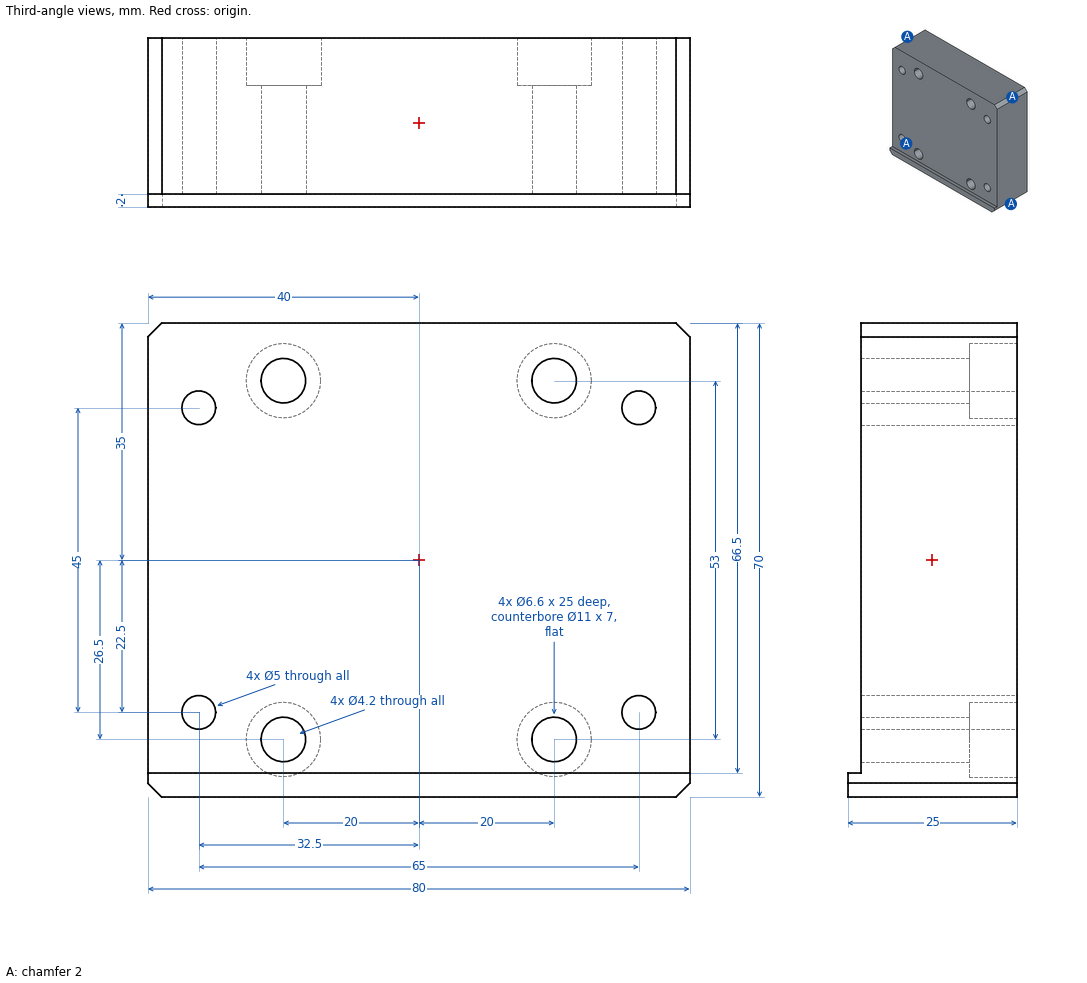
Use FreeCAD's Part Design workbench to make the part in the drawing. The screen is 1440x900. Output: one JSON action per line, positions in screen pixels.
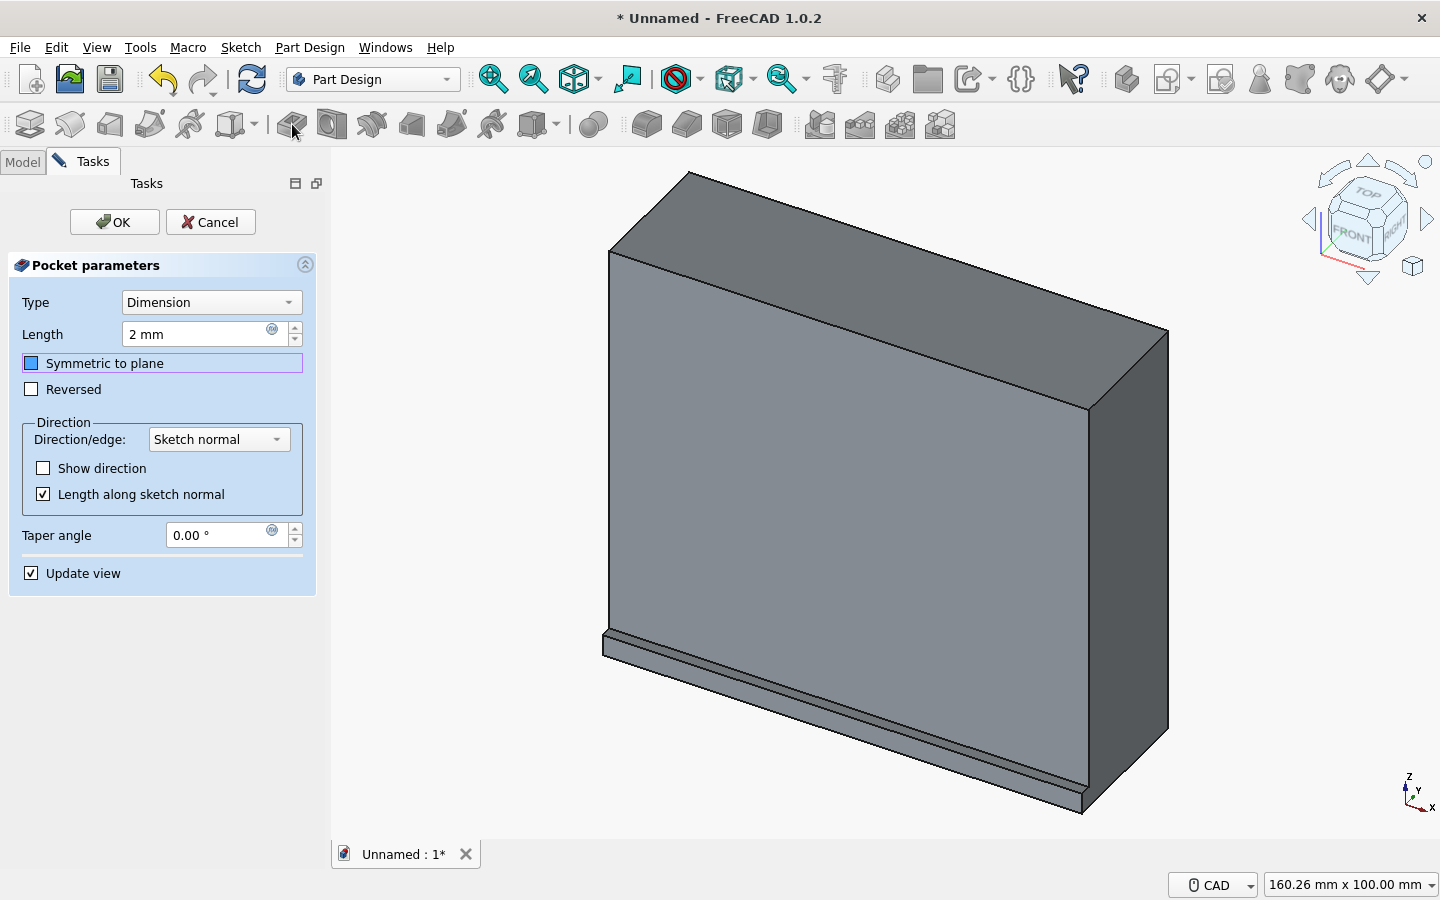
{"action": "left_click", "coordinate": [115, 222]}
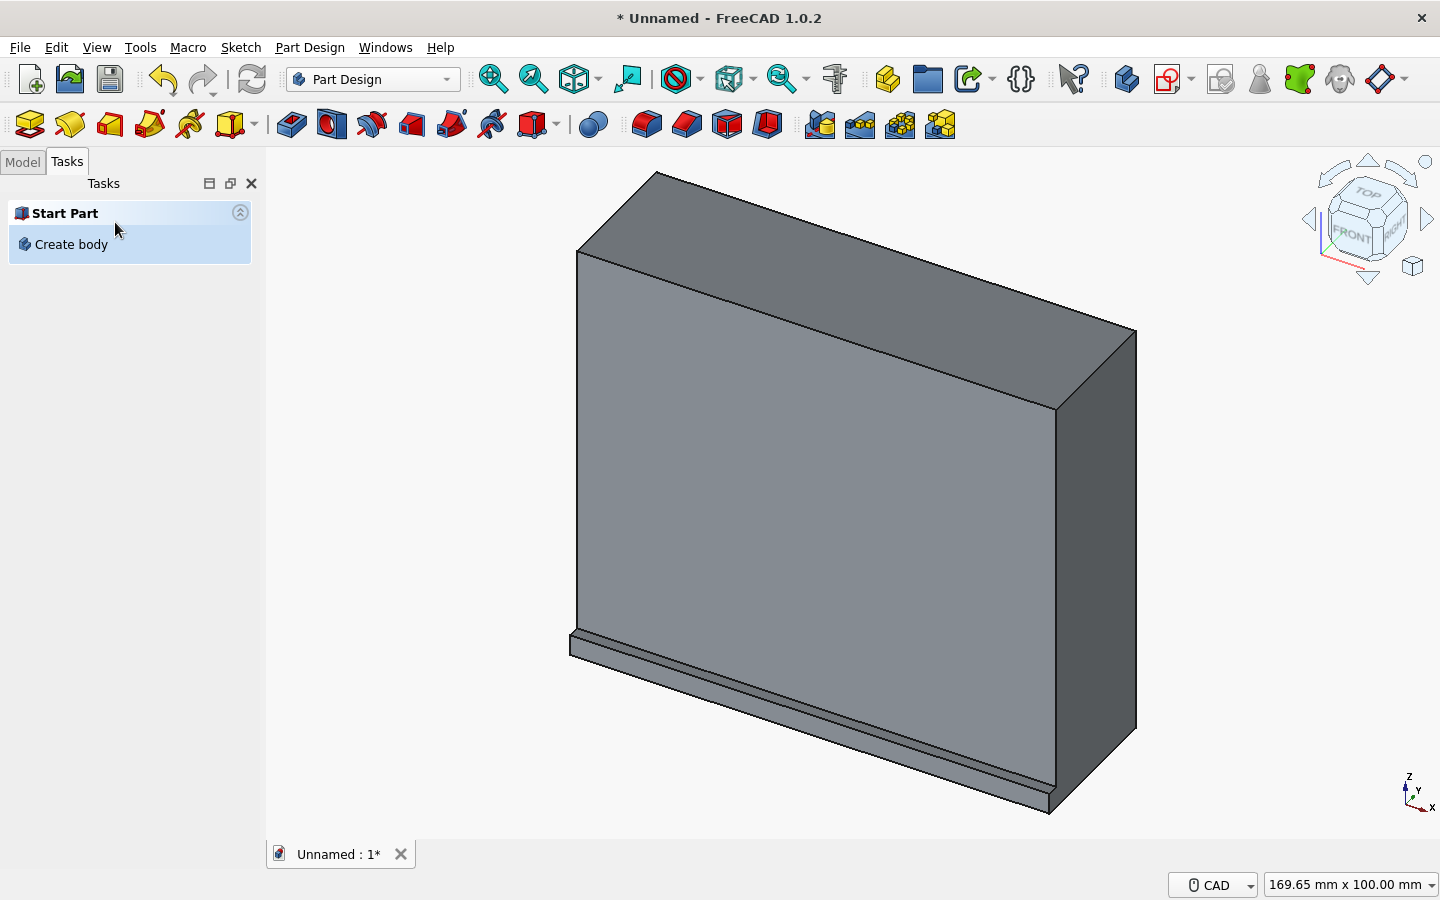
{"action": "left_click", "coordinate": [817, 518]}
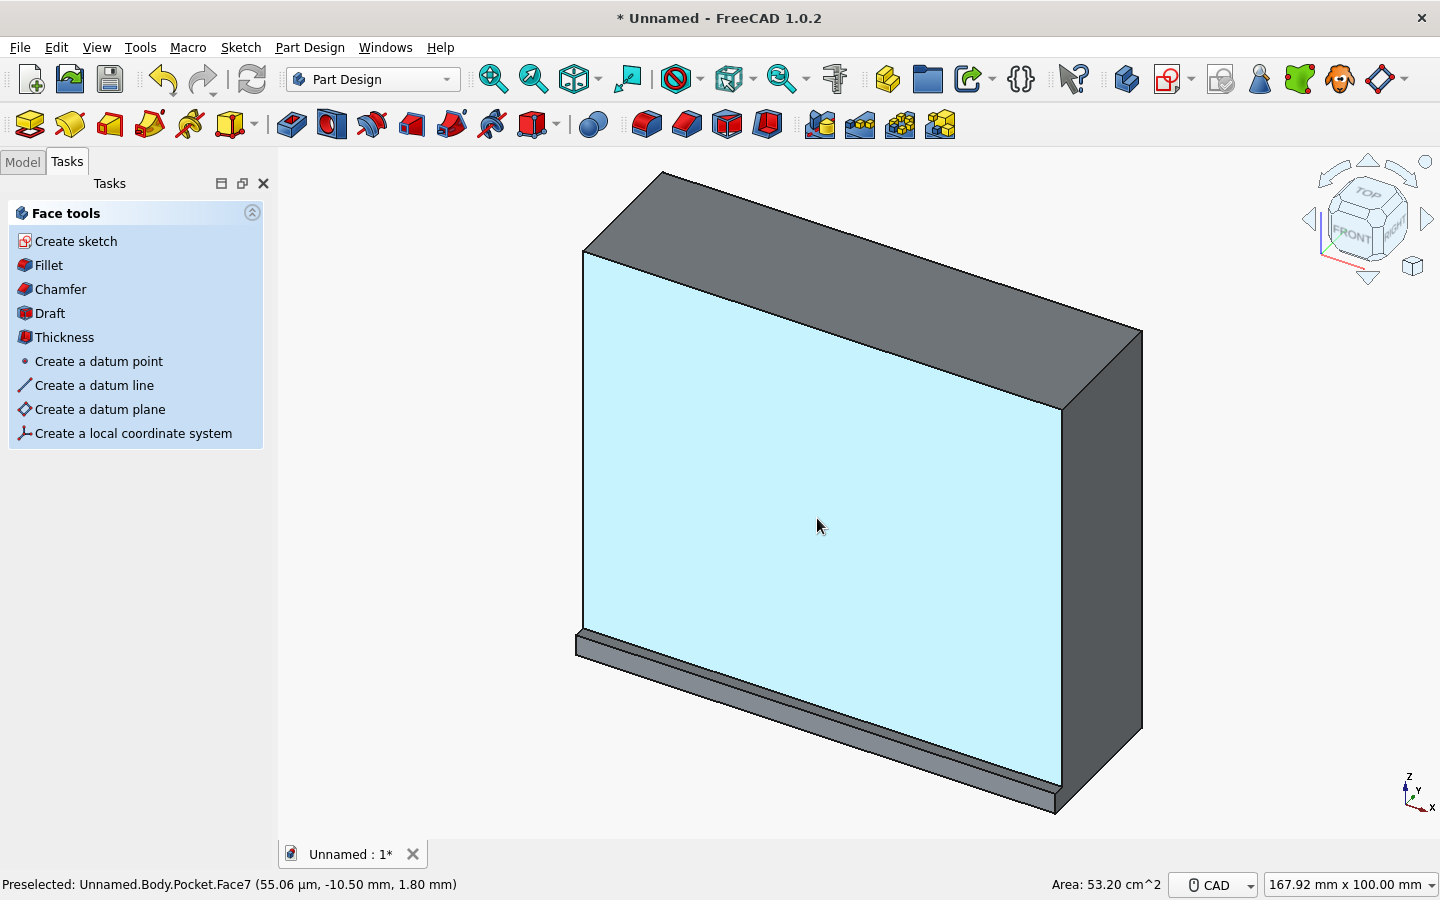
{"action": "left_click", "coordinate": [1168, 80]}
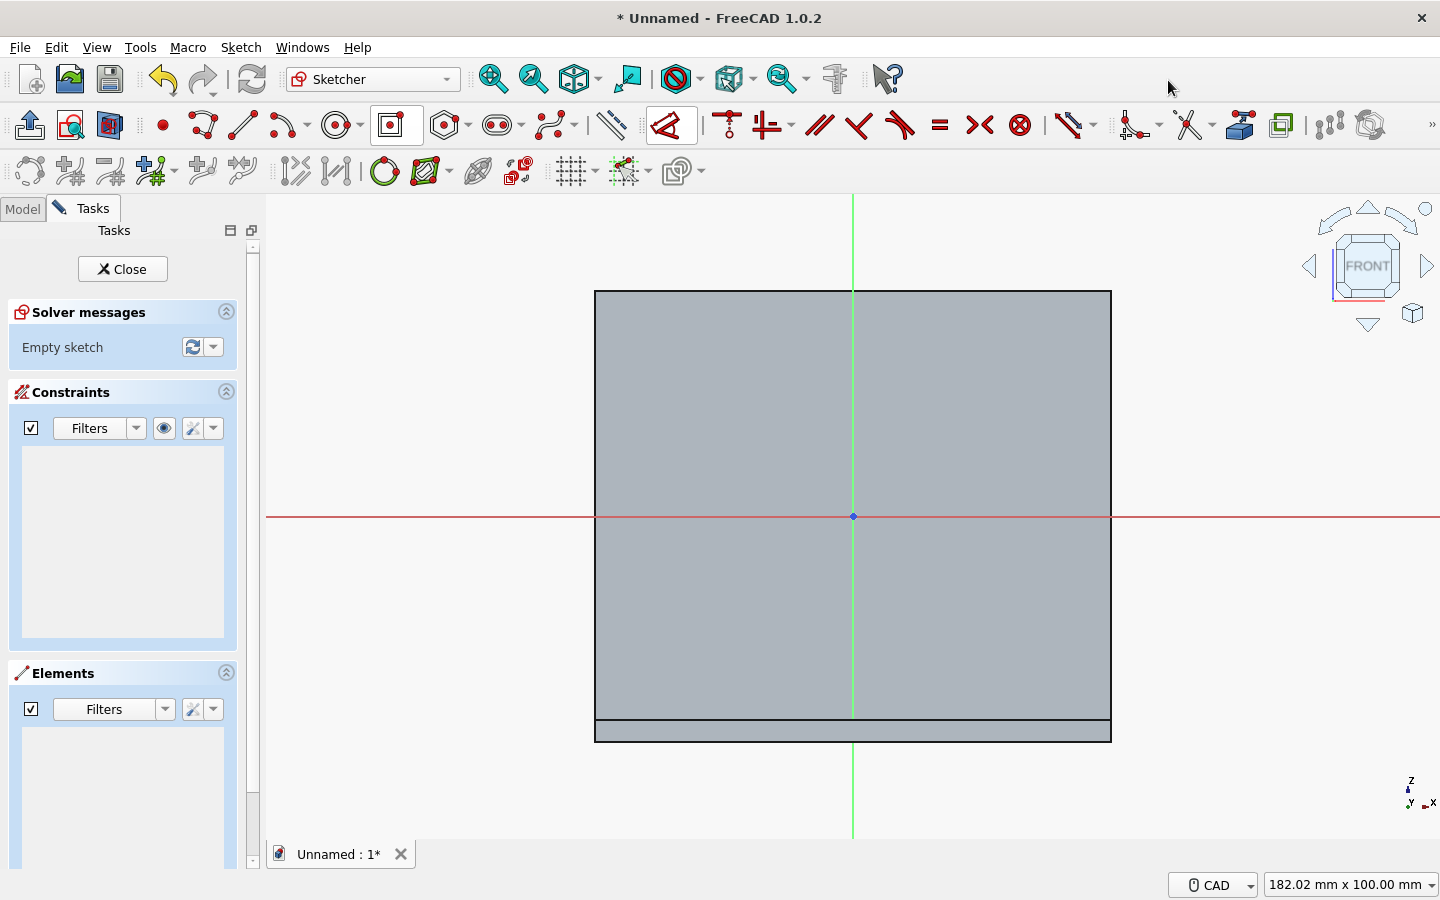
{"action": "left_click", "coordinate": [110, 126]}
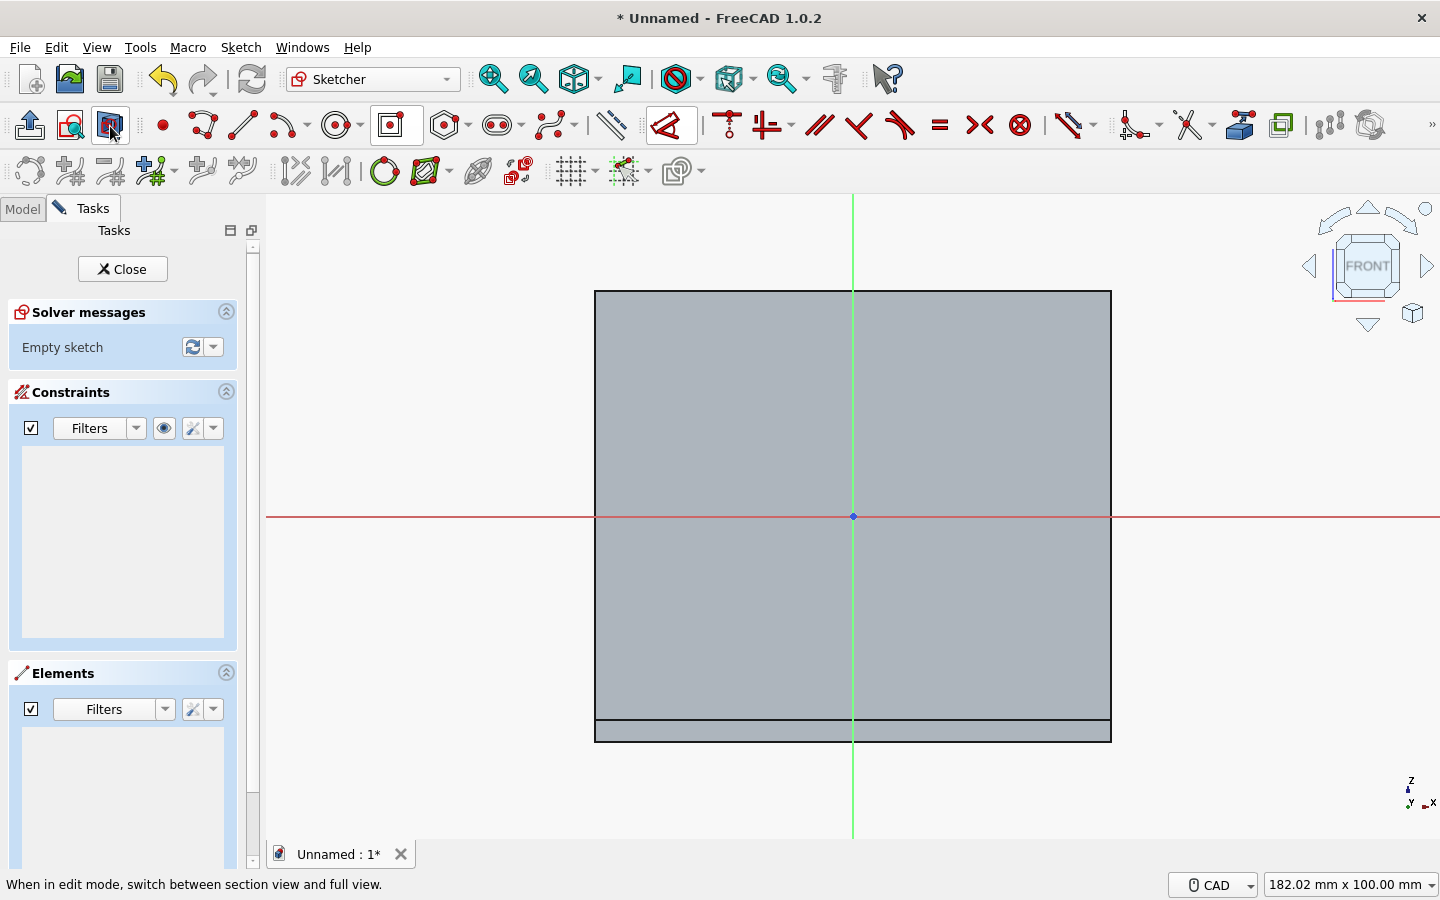
{"action": "left_click", "coordinate": [336, 126]}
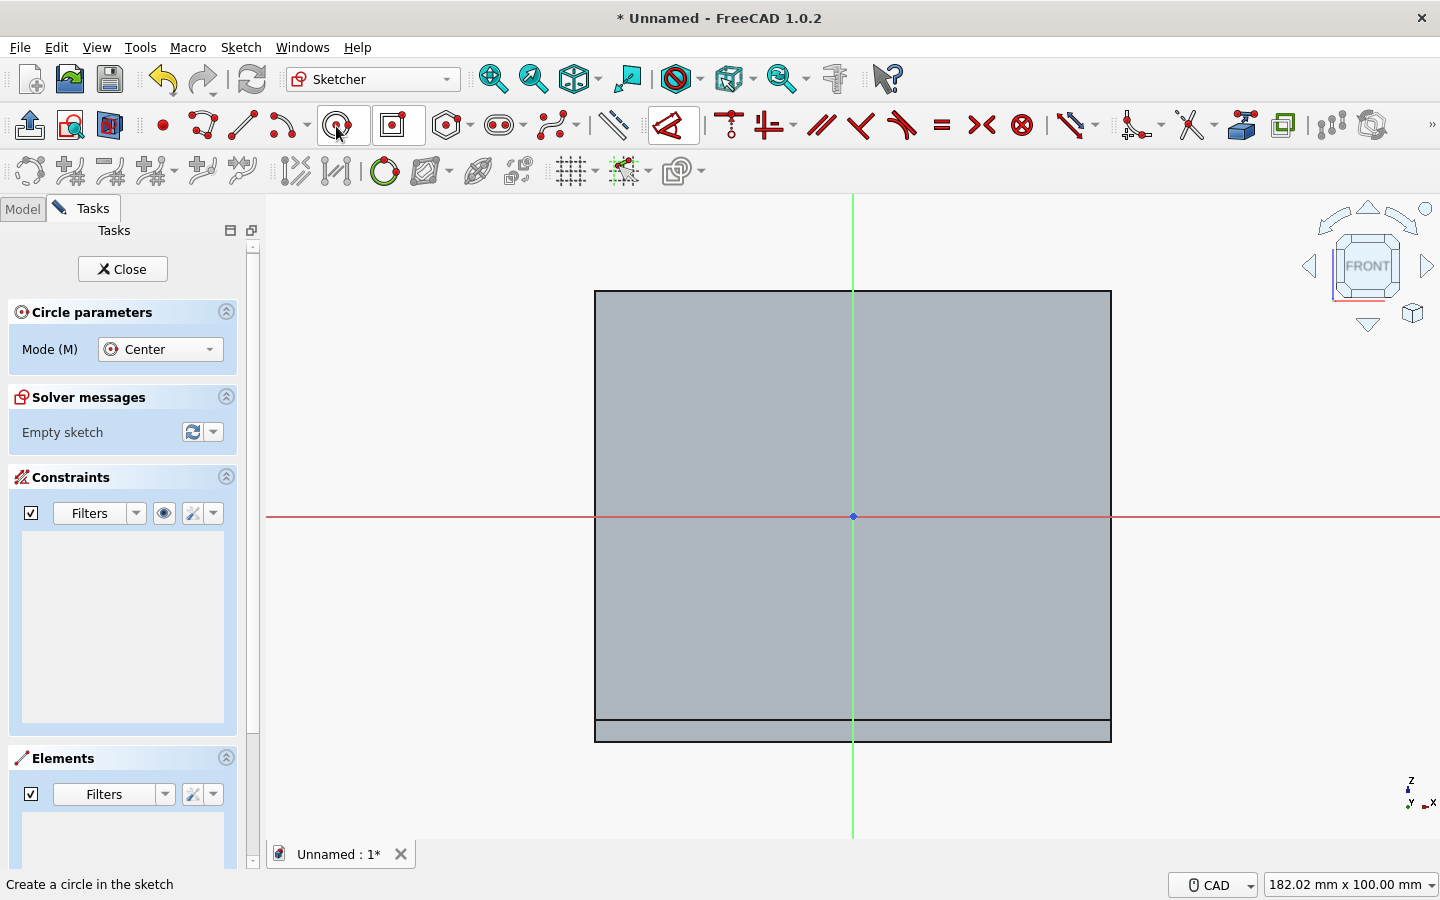
{"action": "scroll", "coordinate": [724, 687], "scroll_direction": "up", "scroll_amount": 3}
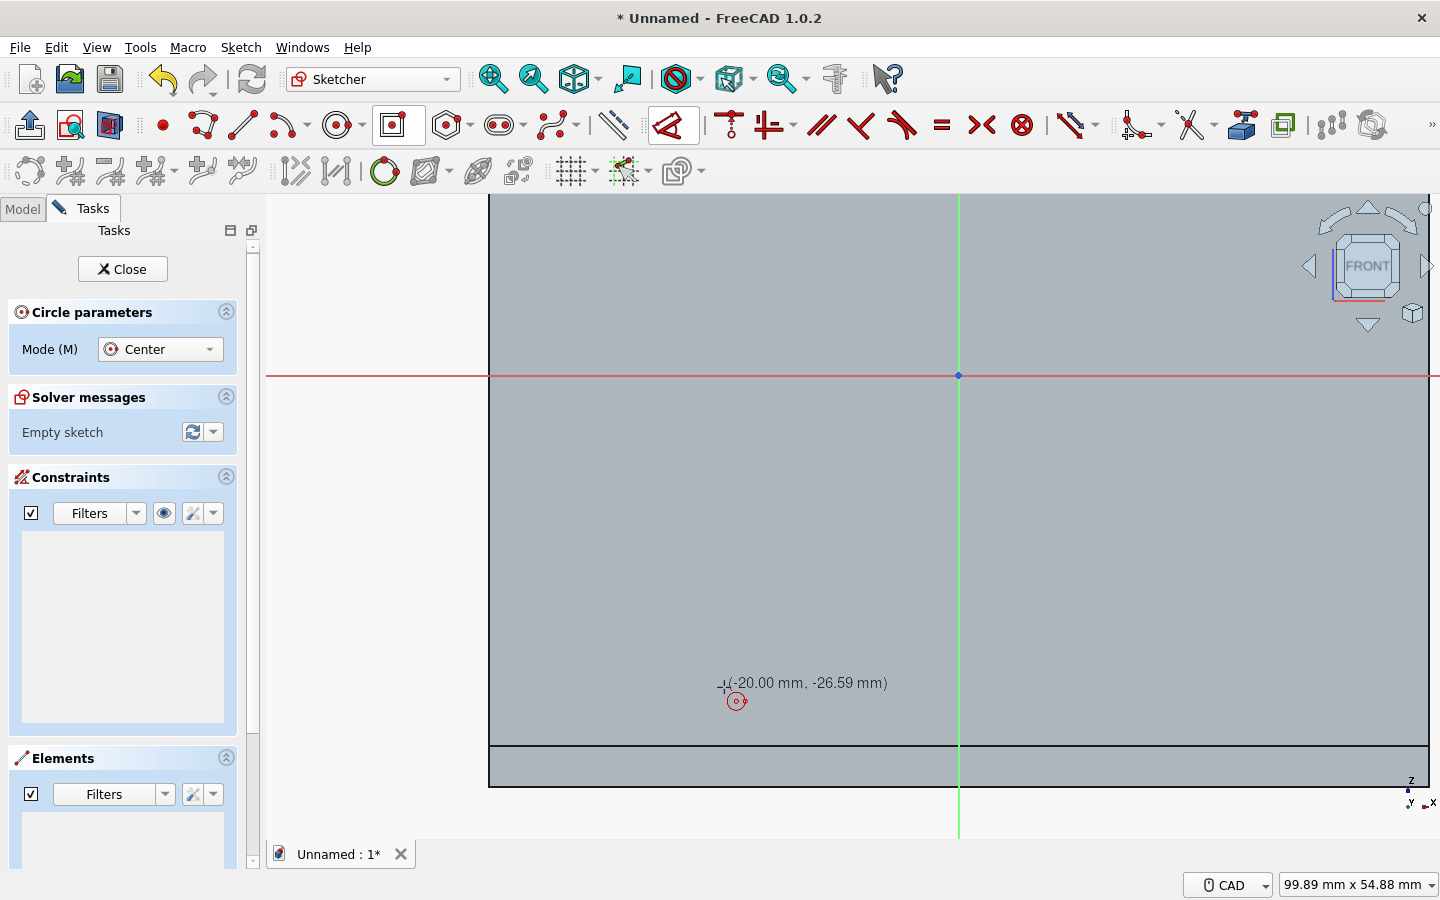
{"action": "left_click", "coordinate": [724, 687]}
{"action": "mouse_move", "coordinate": [741, 670]}